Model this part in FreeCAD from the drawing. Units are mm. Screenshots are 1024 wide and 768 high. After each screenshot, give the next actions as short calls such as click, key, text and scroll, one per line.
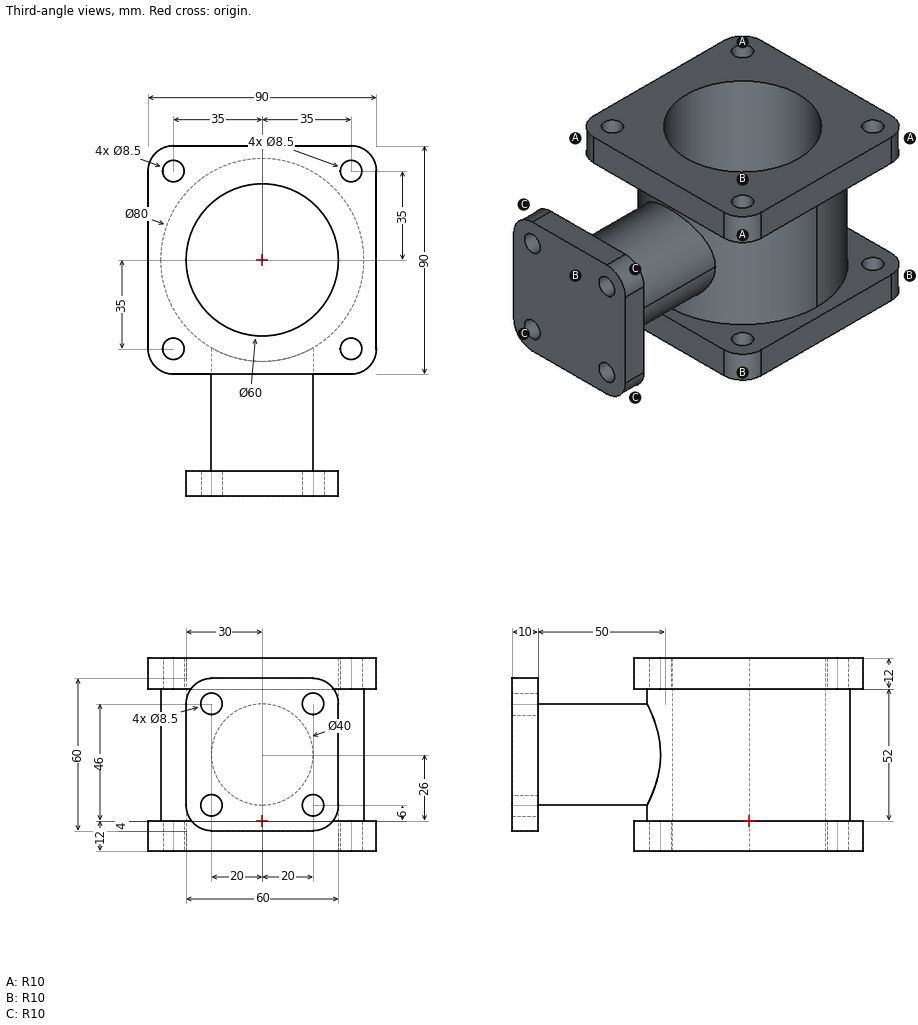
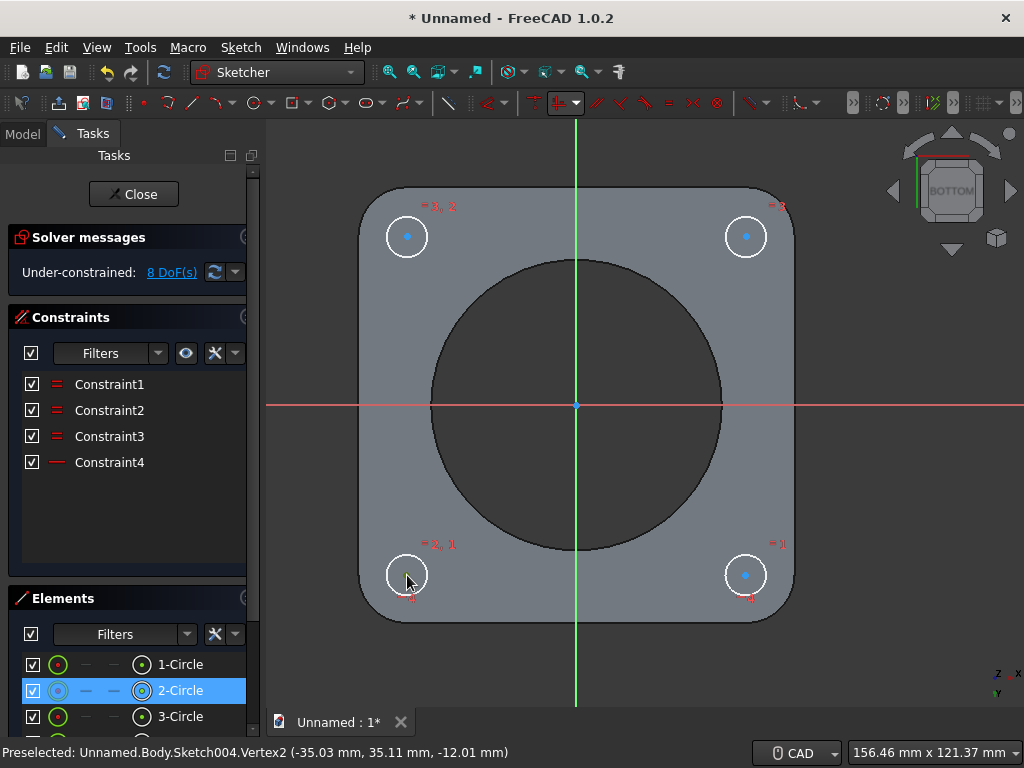
click(407, 237)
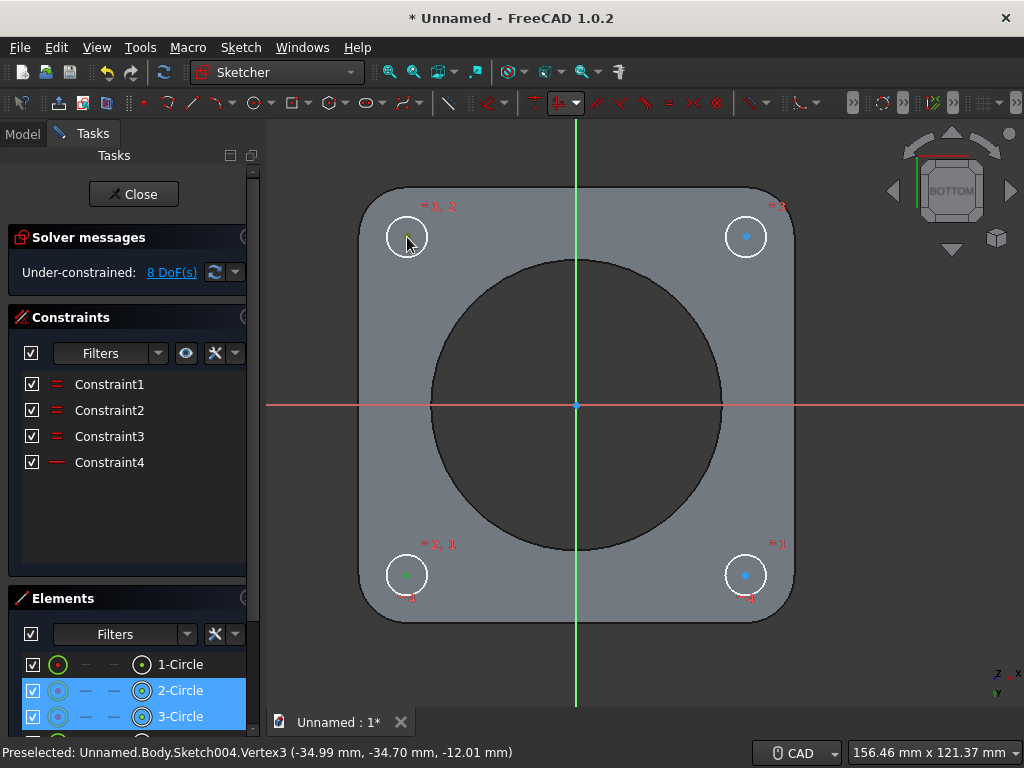
click(578, 104)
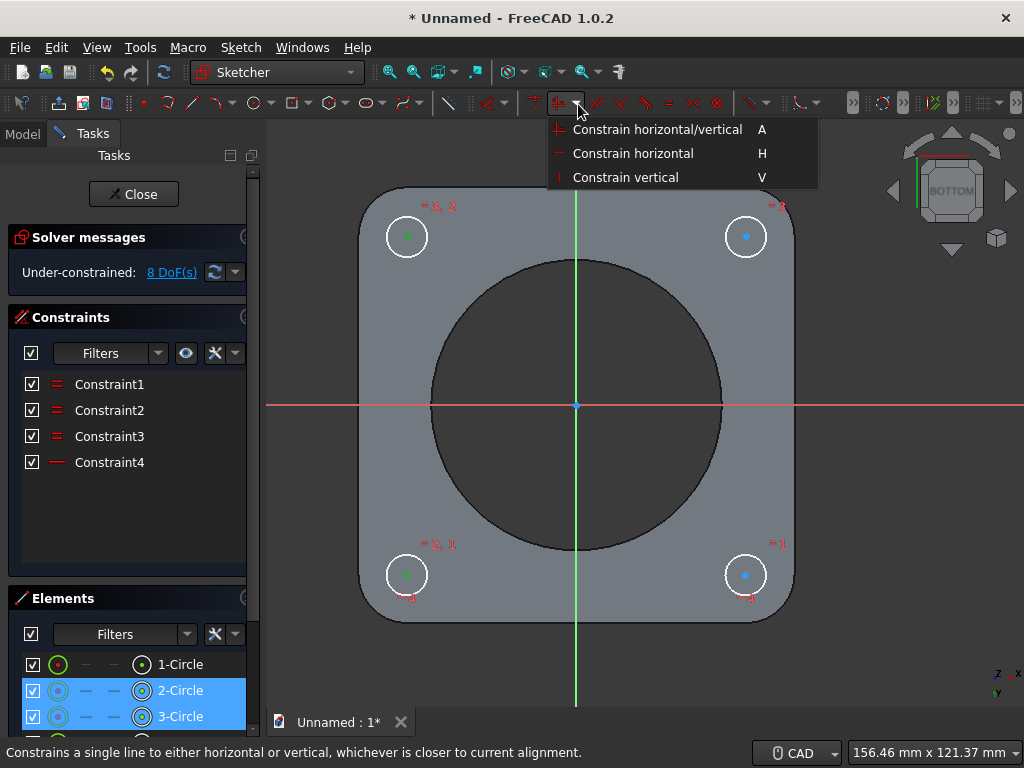
click(683, 177)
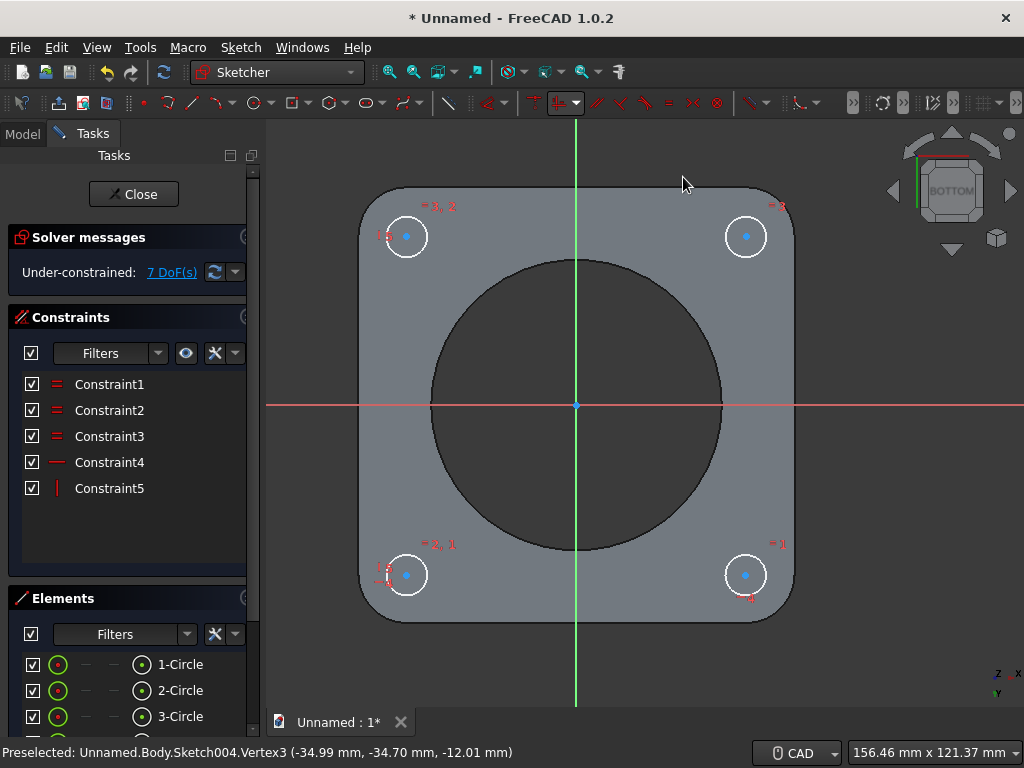
click(746, 575)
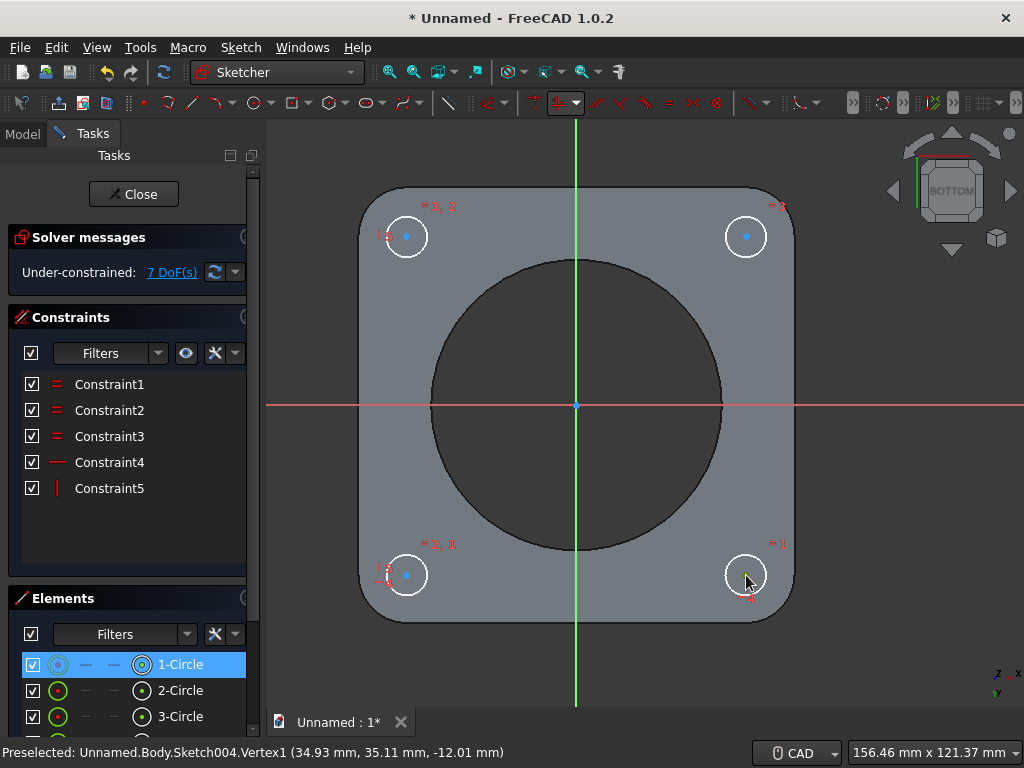
click(746, 237)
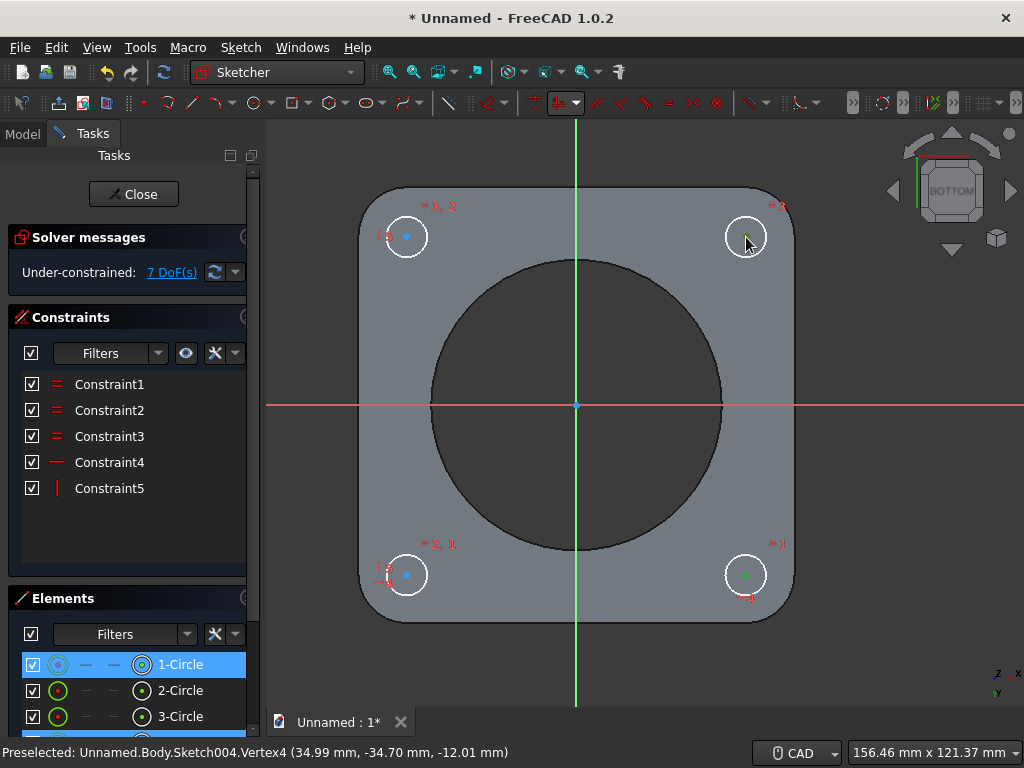
click(578, 104)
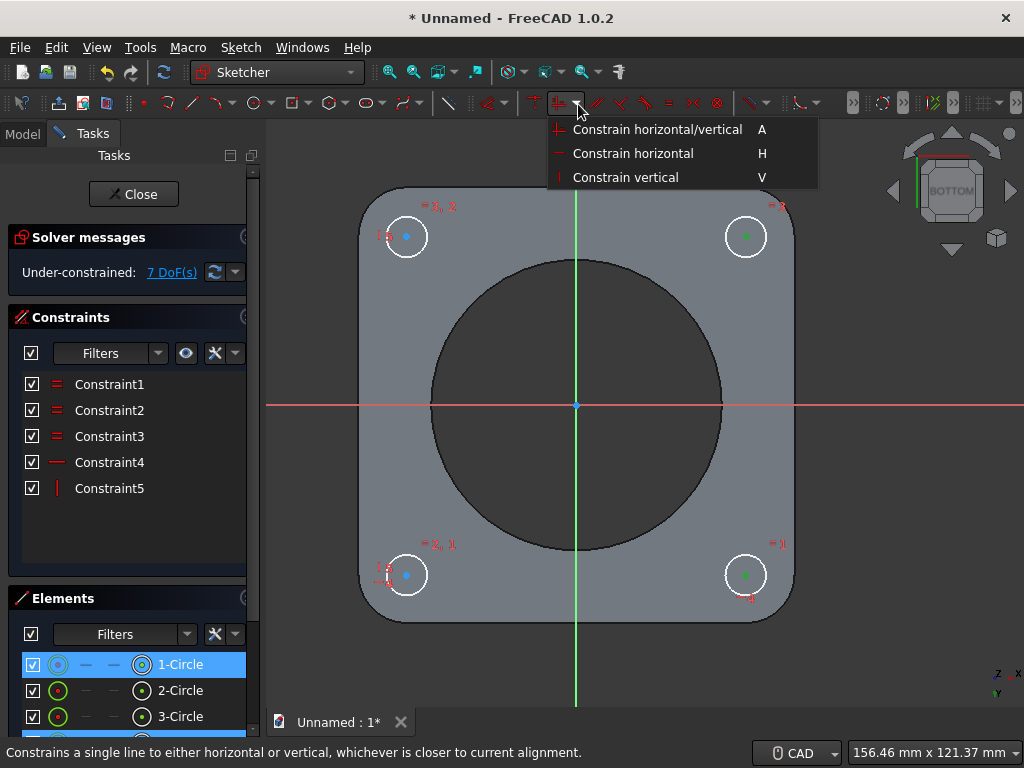
click(683, 177)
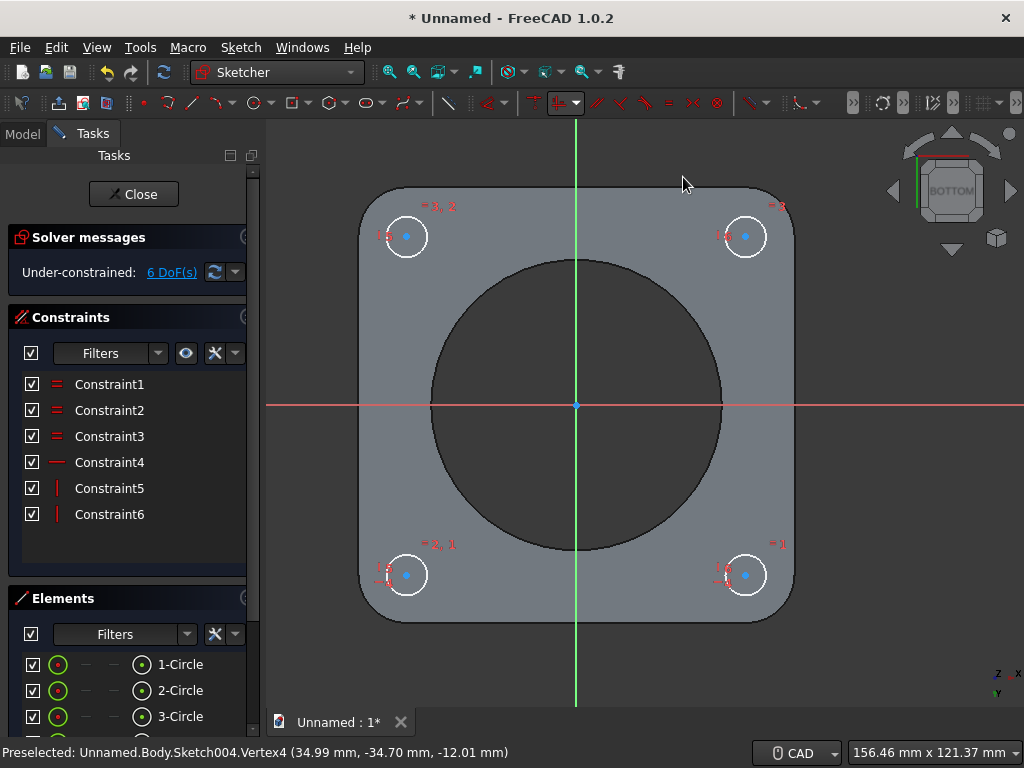
click(407, 237)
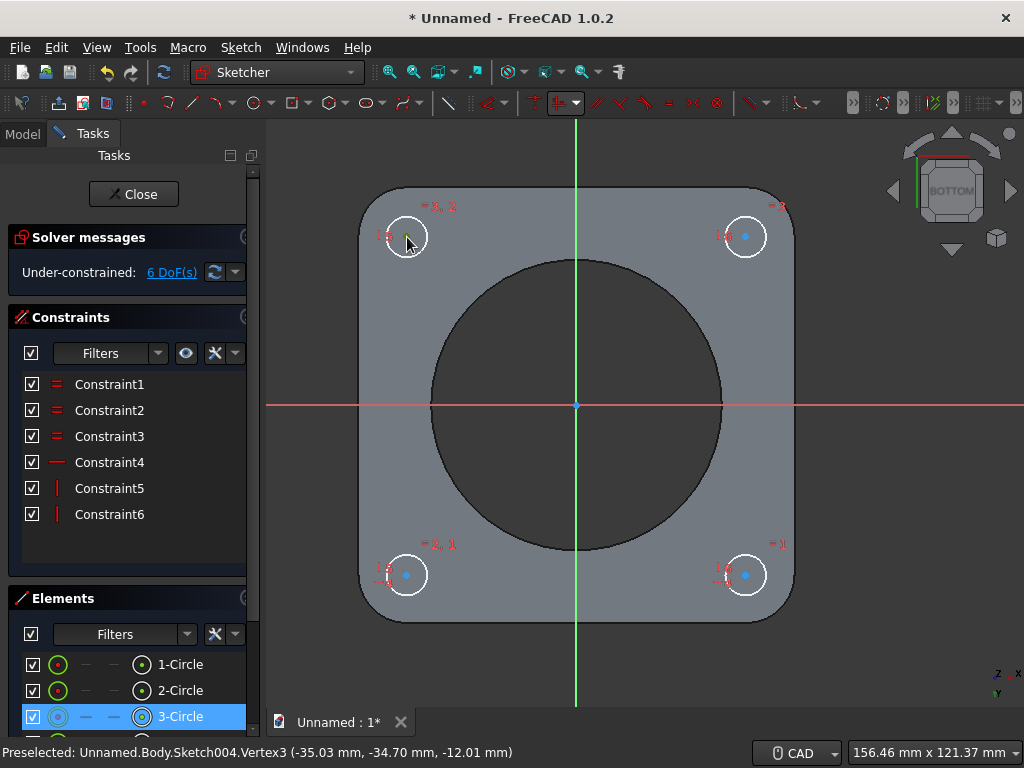
click(746, 237)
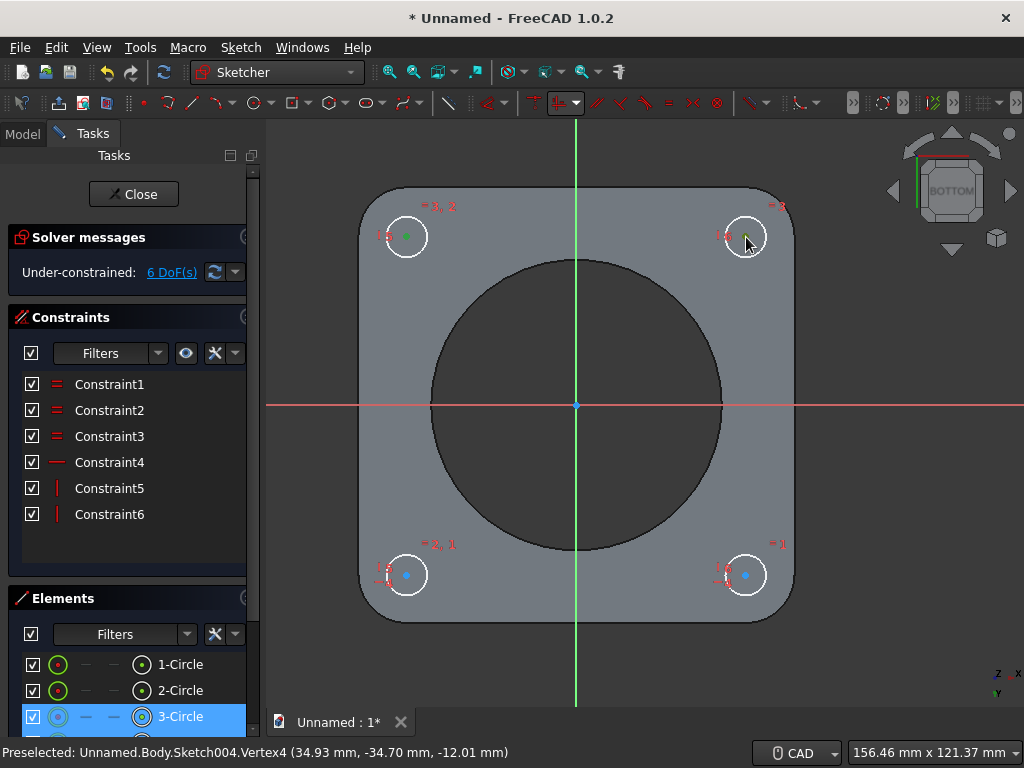
click(578, 104)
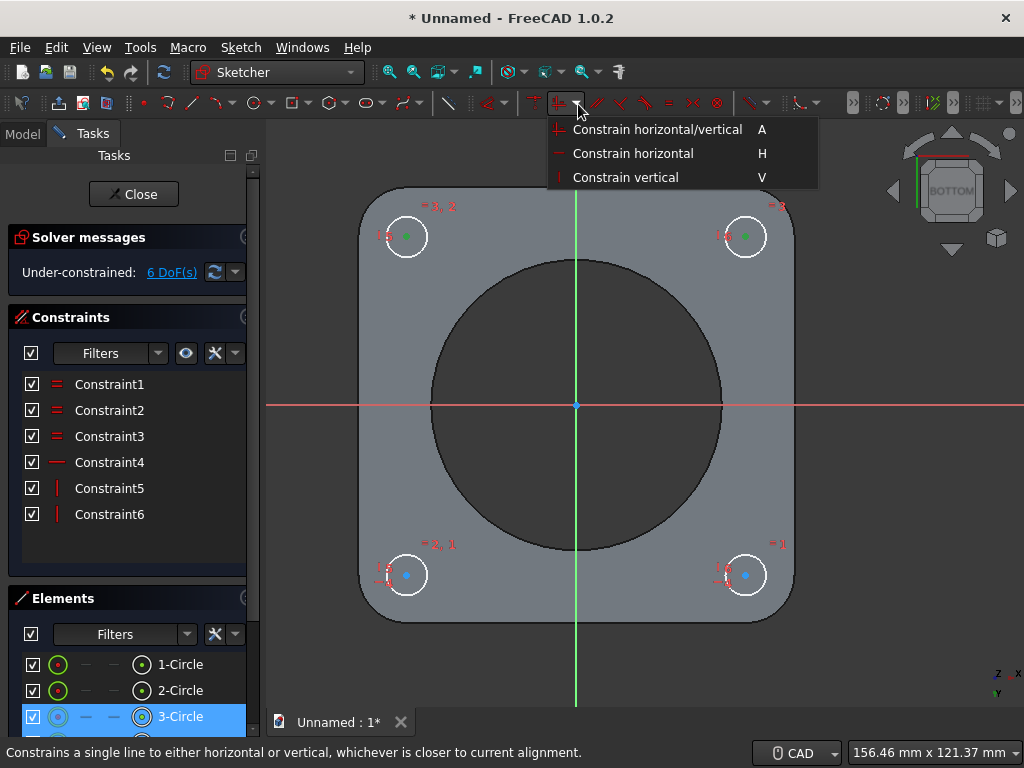
click(683, 153)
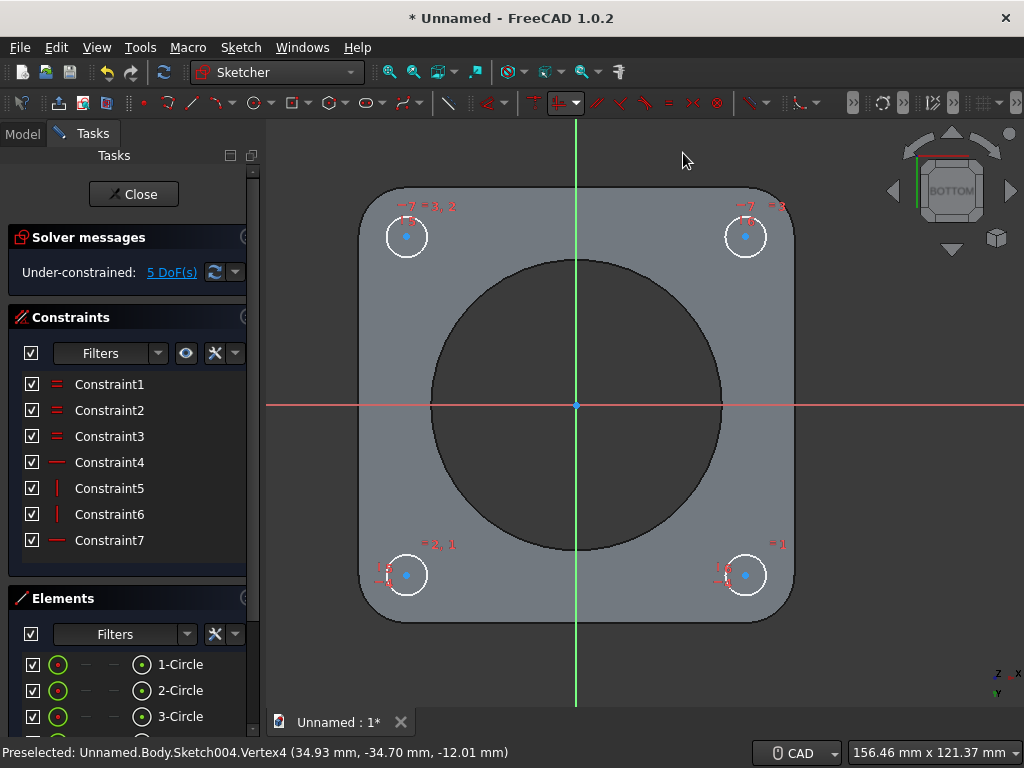
key(d)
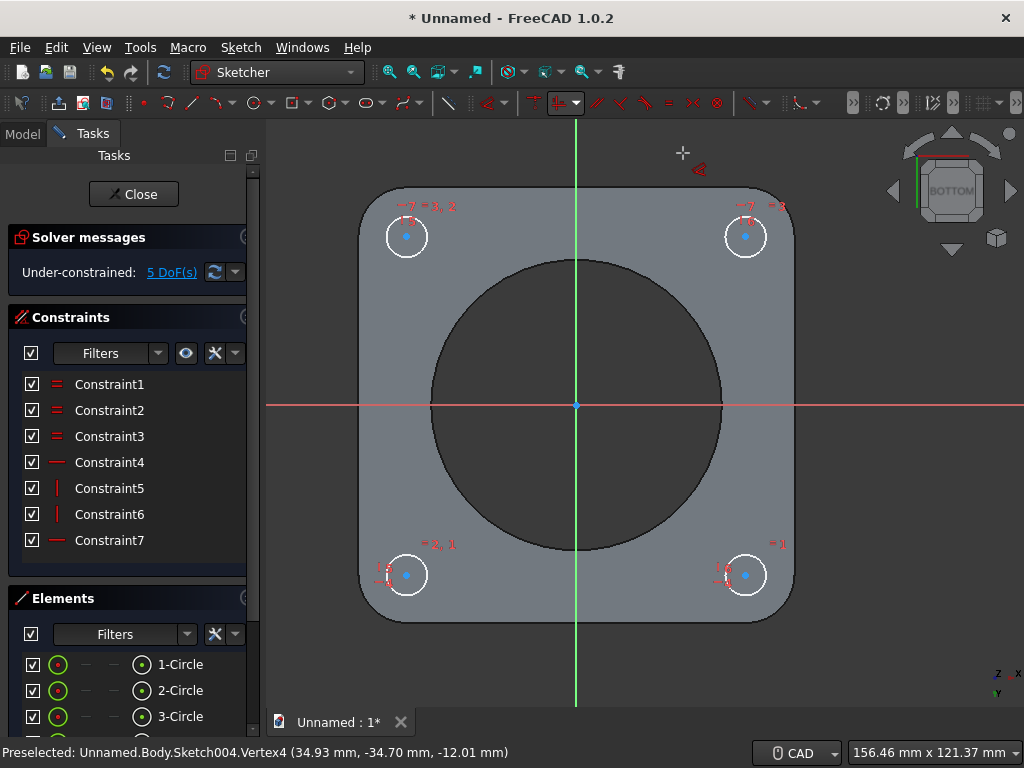
click(760, 561)
click(783, 538)